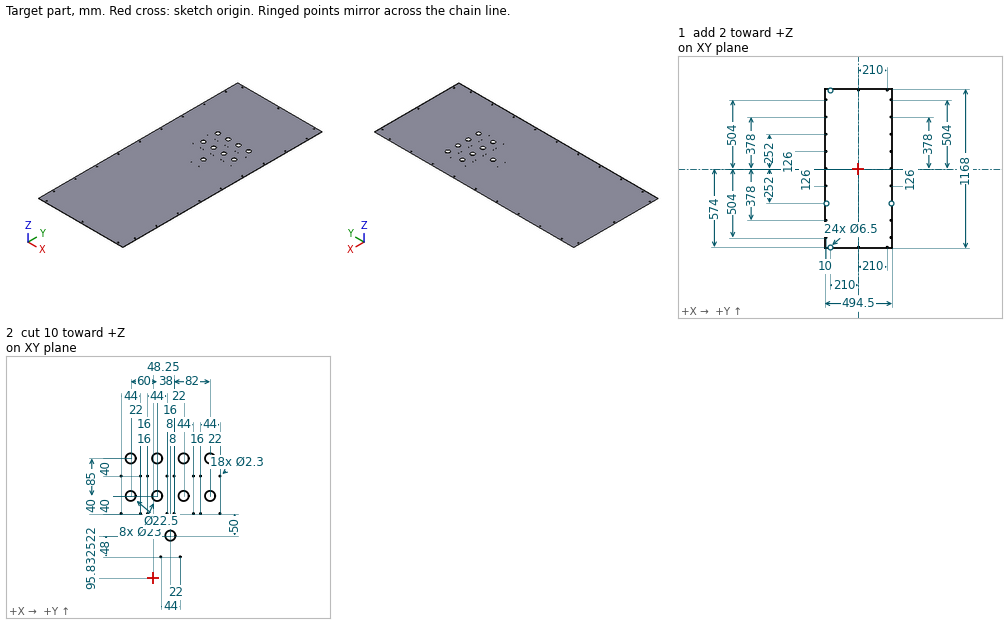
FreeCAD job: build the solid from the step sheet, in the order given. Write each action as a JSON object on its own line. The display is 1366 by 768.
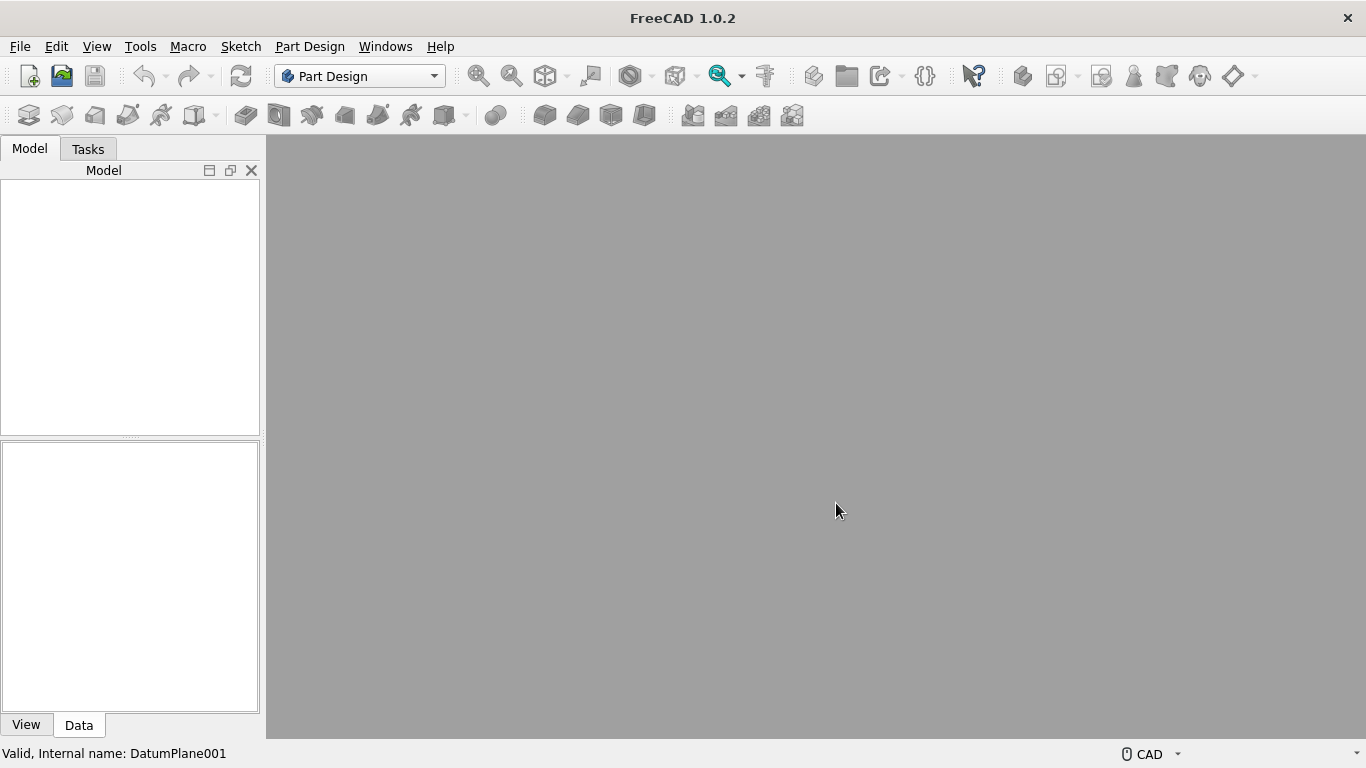
{"action": "left_click", "coordinate": [29, 76]}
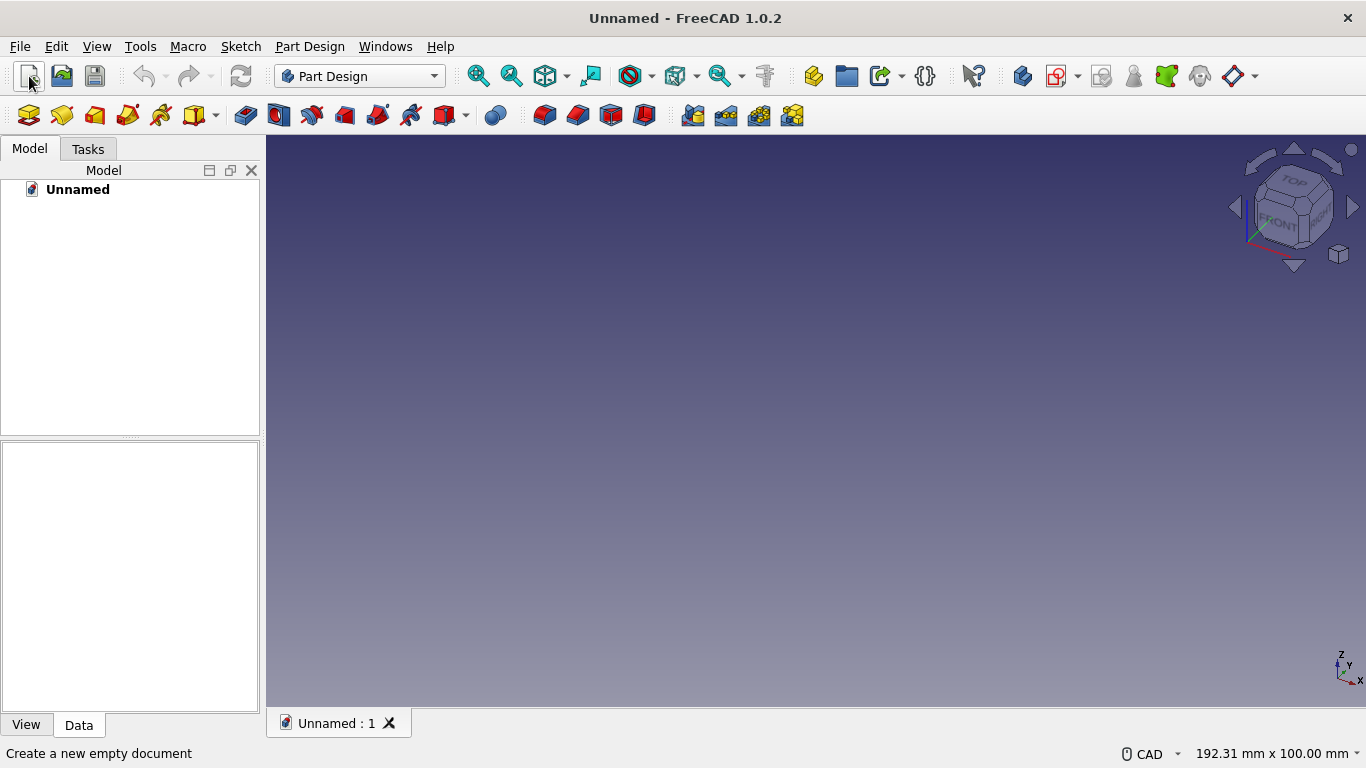
{"action": "left_click", "coordinate": [1056, 76]}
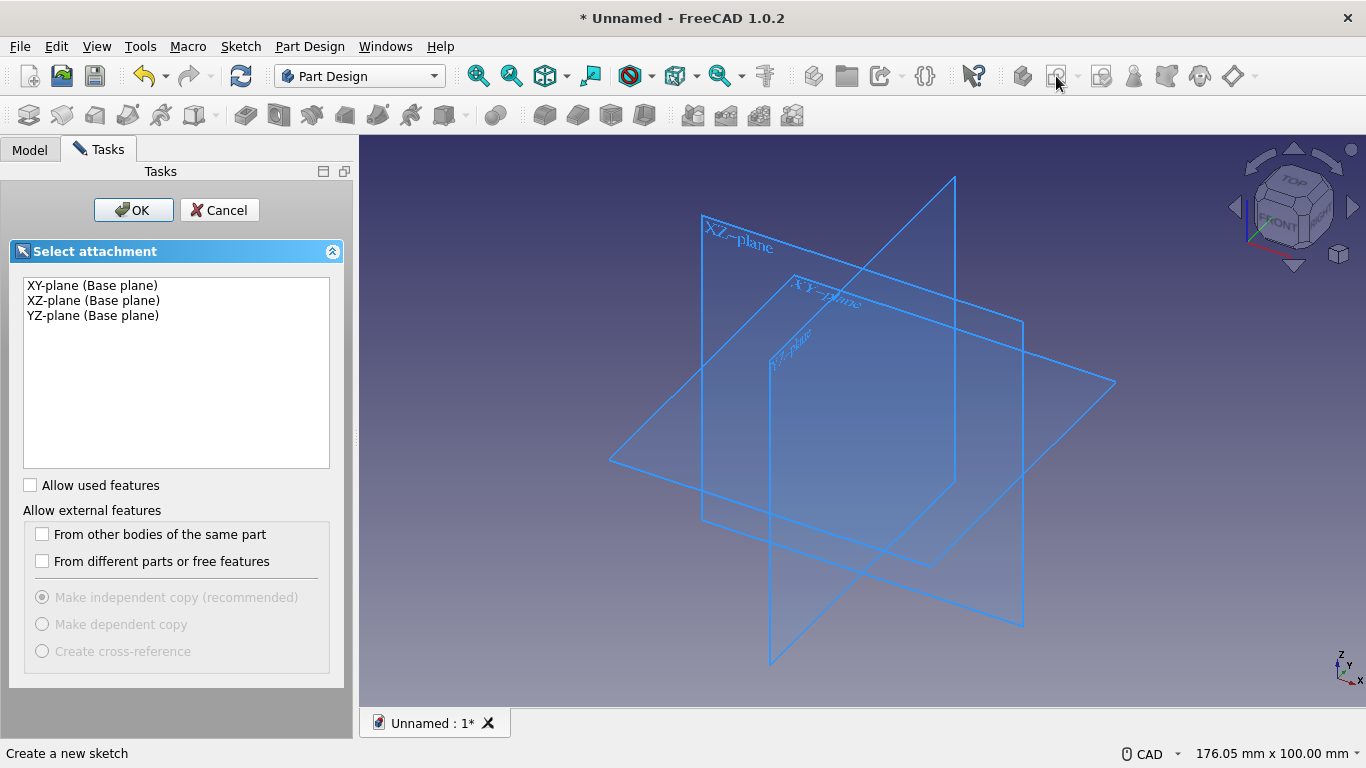
{"action": "left_click", "coordinate": [84, 286]}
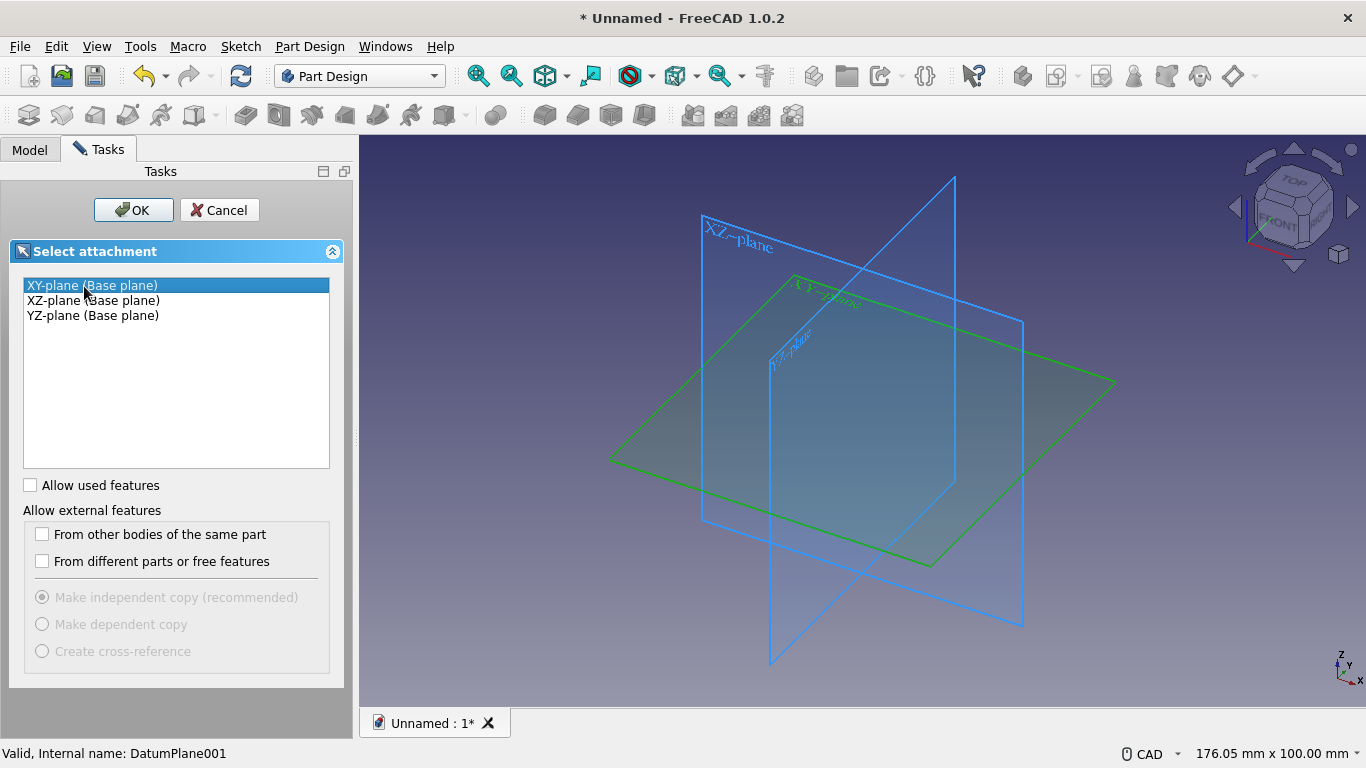
{"action": "left_click", "coordinate": [134, 210]}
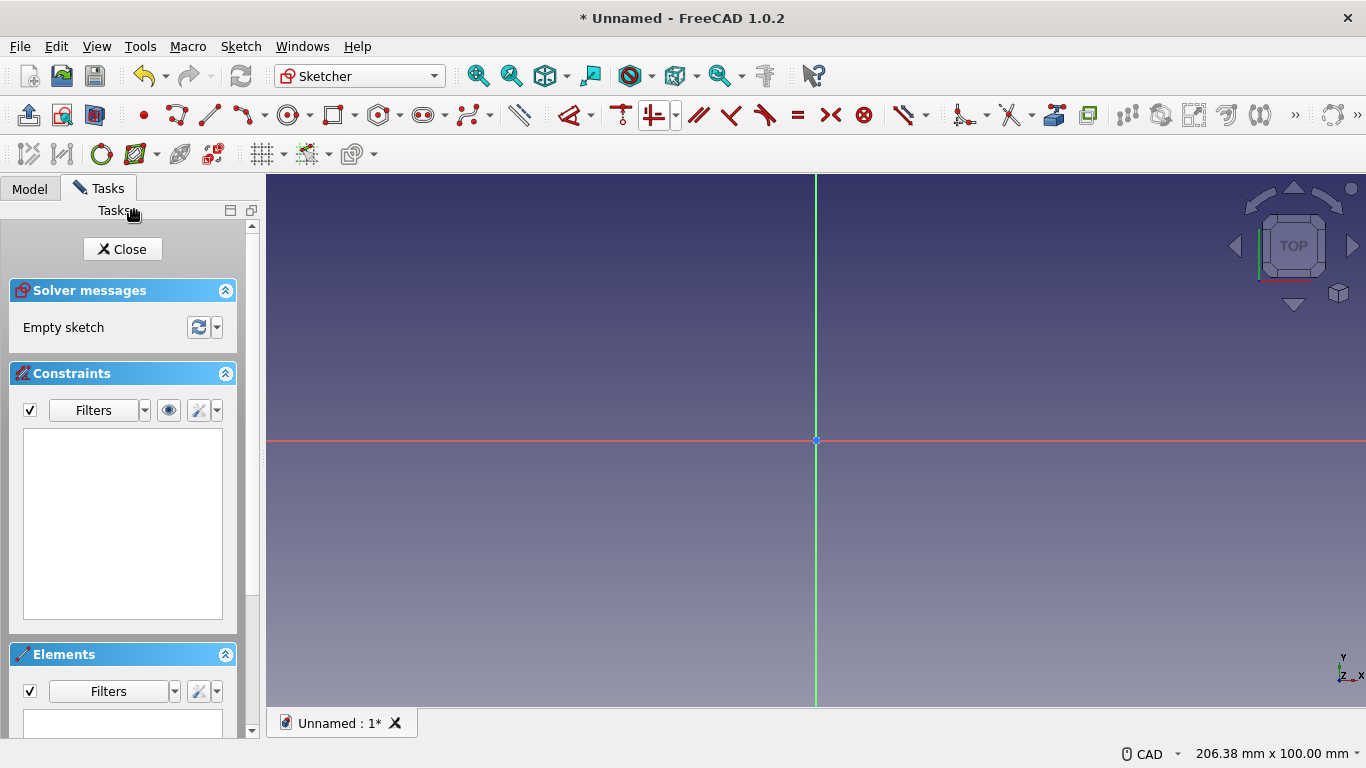
{"action": "scroll", "coordinate": [744, 440], "scroll_direction": "down", "scroll_amount": 15}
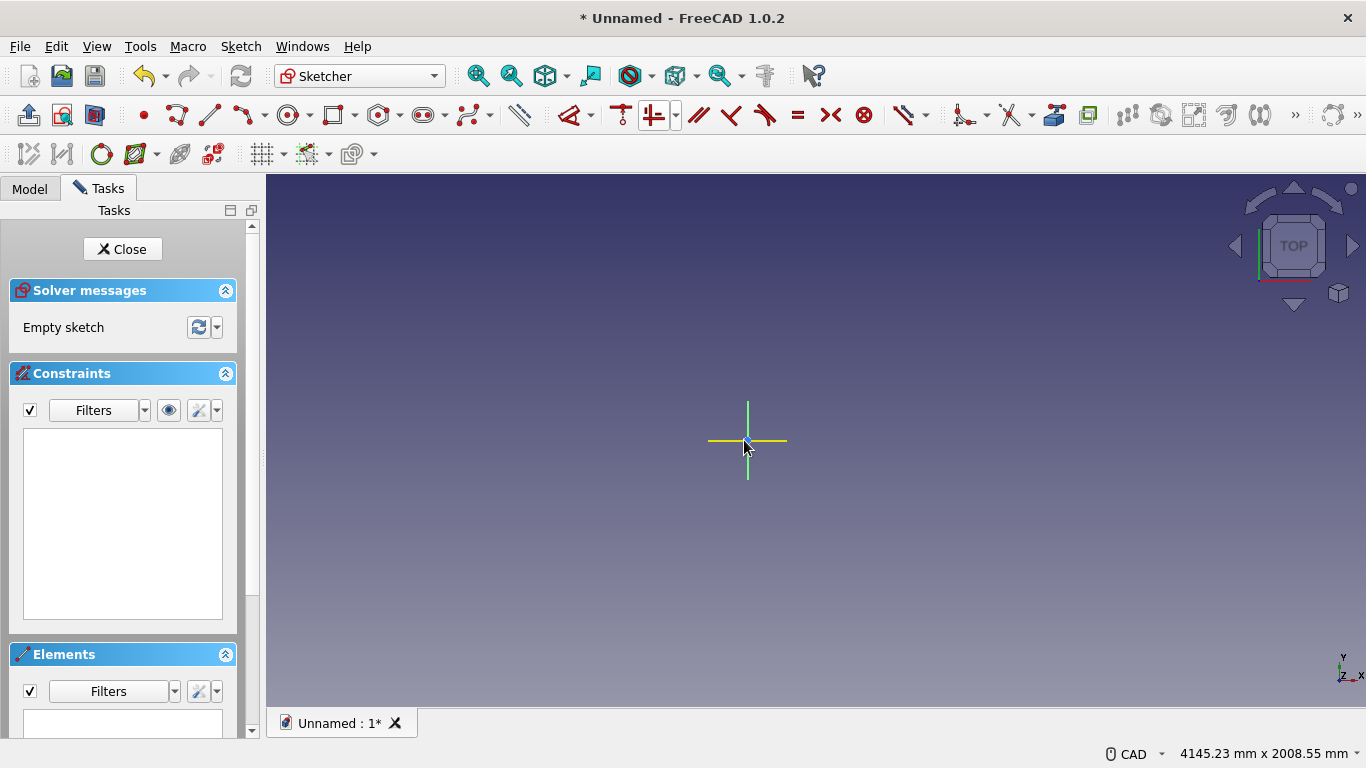
{"action": "left_click", "coordinate": [354, 116]}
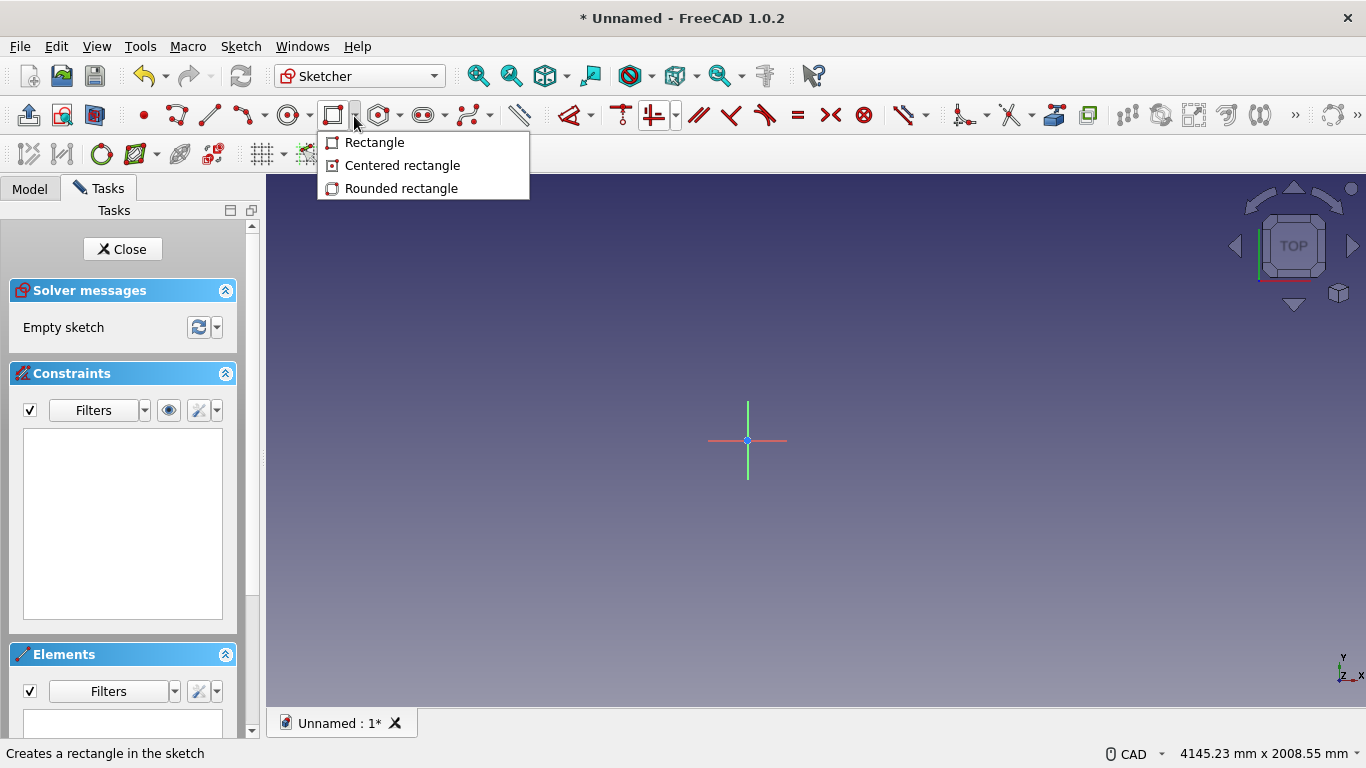
{"action": "left_click", "coordinate": [424, 166]}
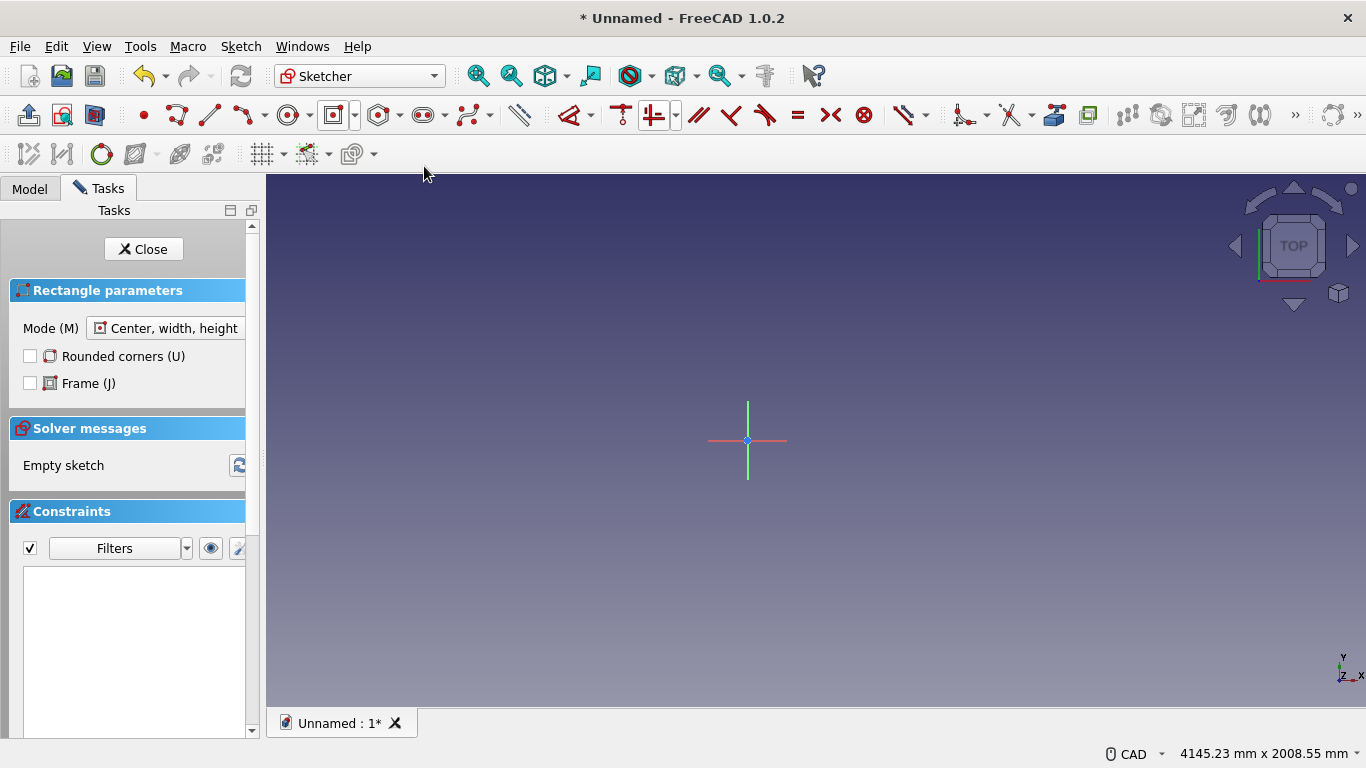
{"action": "left_click", "coordinate": [748, 440]}
{"action": "mouse_move", "coordinate": [814, 286]}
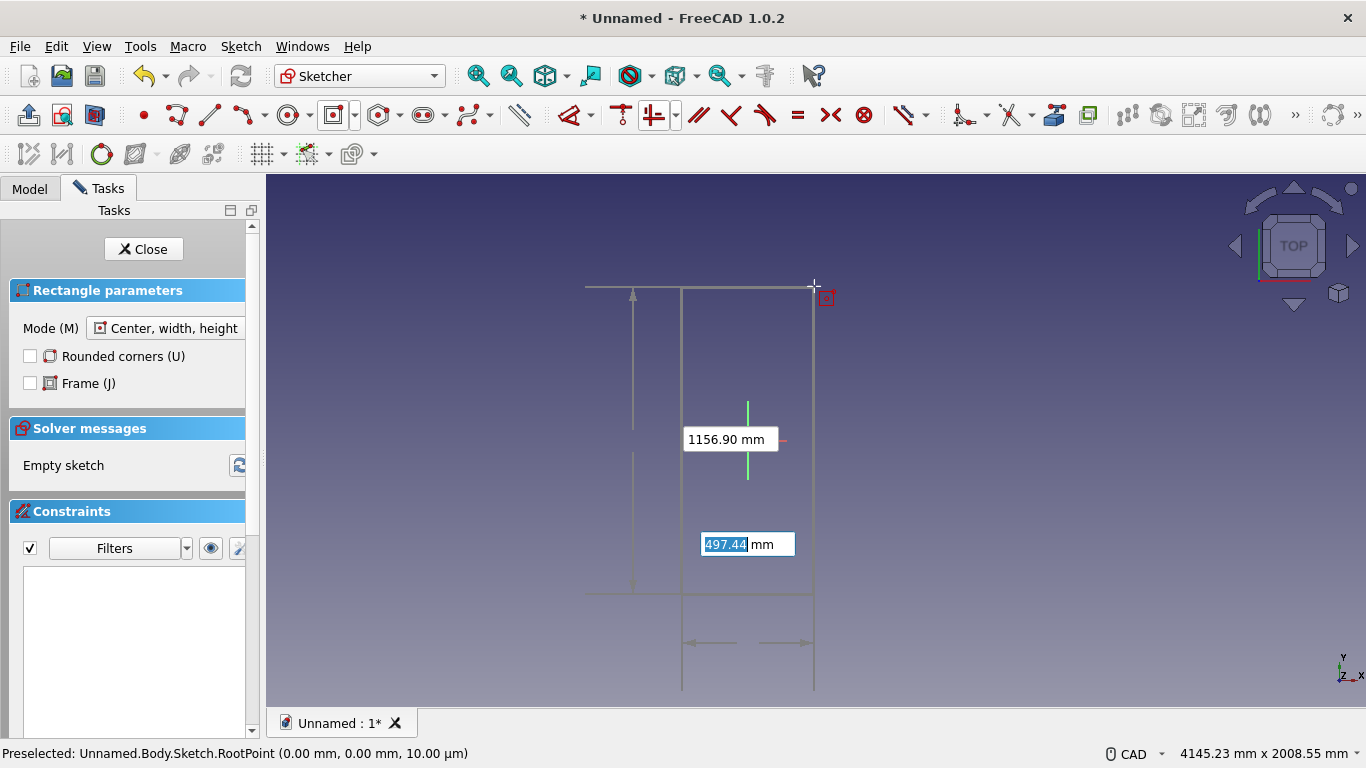
{"action": "type", "text": "494.5"}
{"action": "key", "text": "Tab"}
{"action": "type", "text": "1168"}
{"action": "key", "text": "Return"}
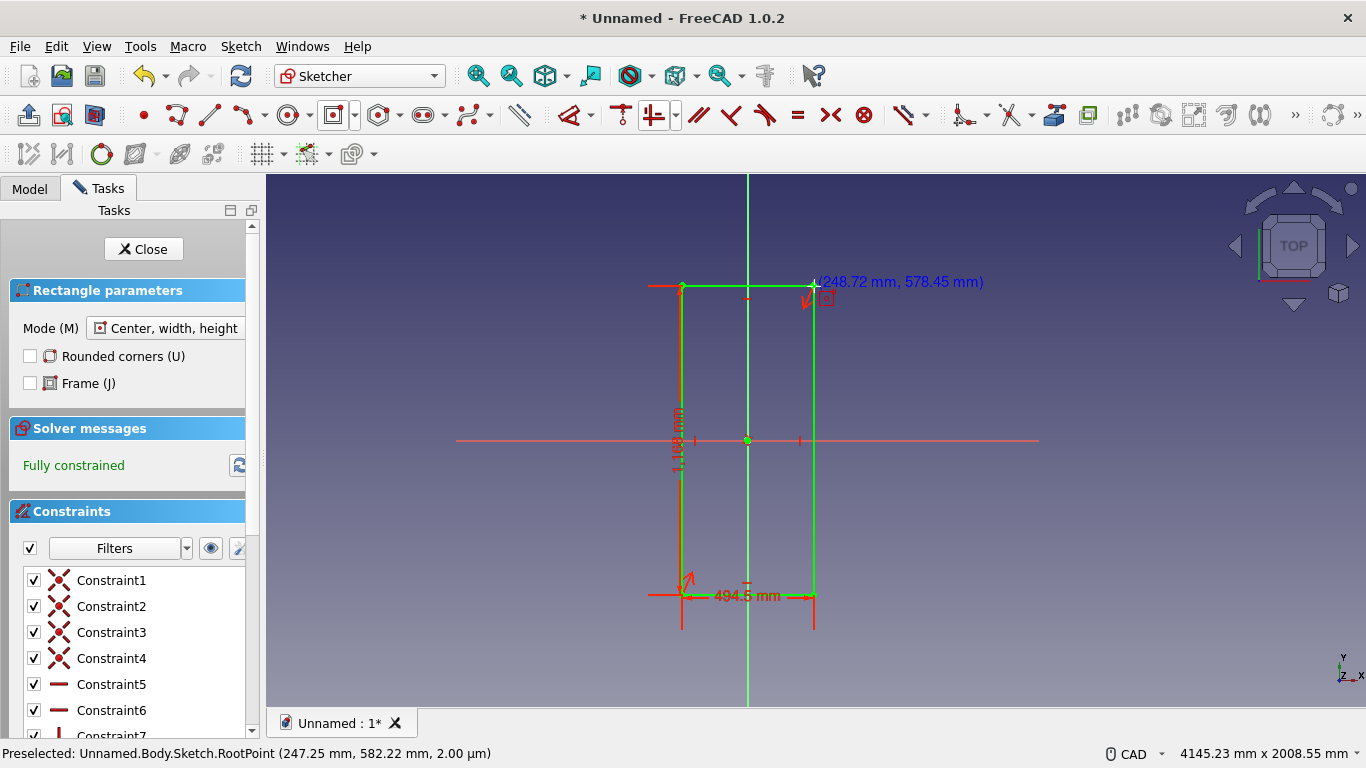
{"action": "left_click", "coordinate": [288, 116]}